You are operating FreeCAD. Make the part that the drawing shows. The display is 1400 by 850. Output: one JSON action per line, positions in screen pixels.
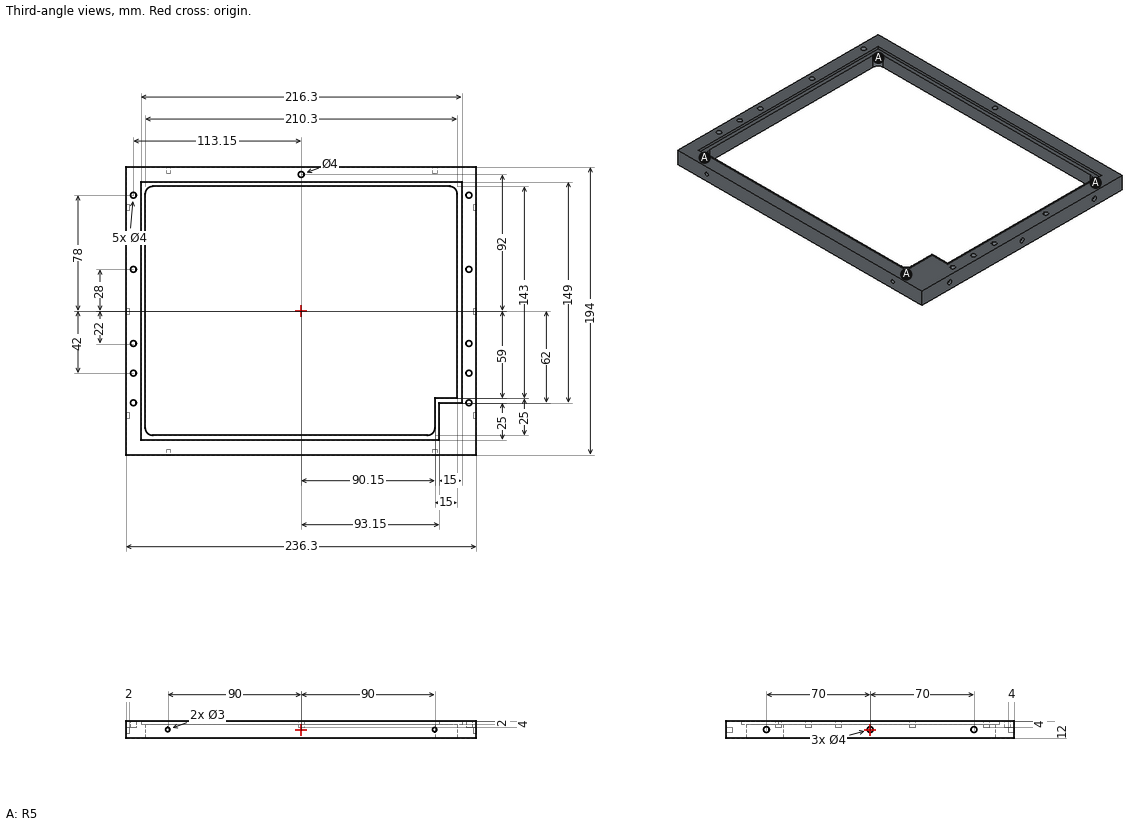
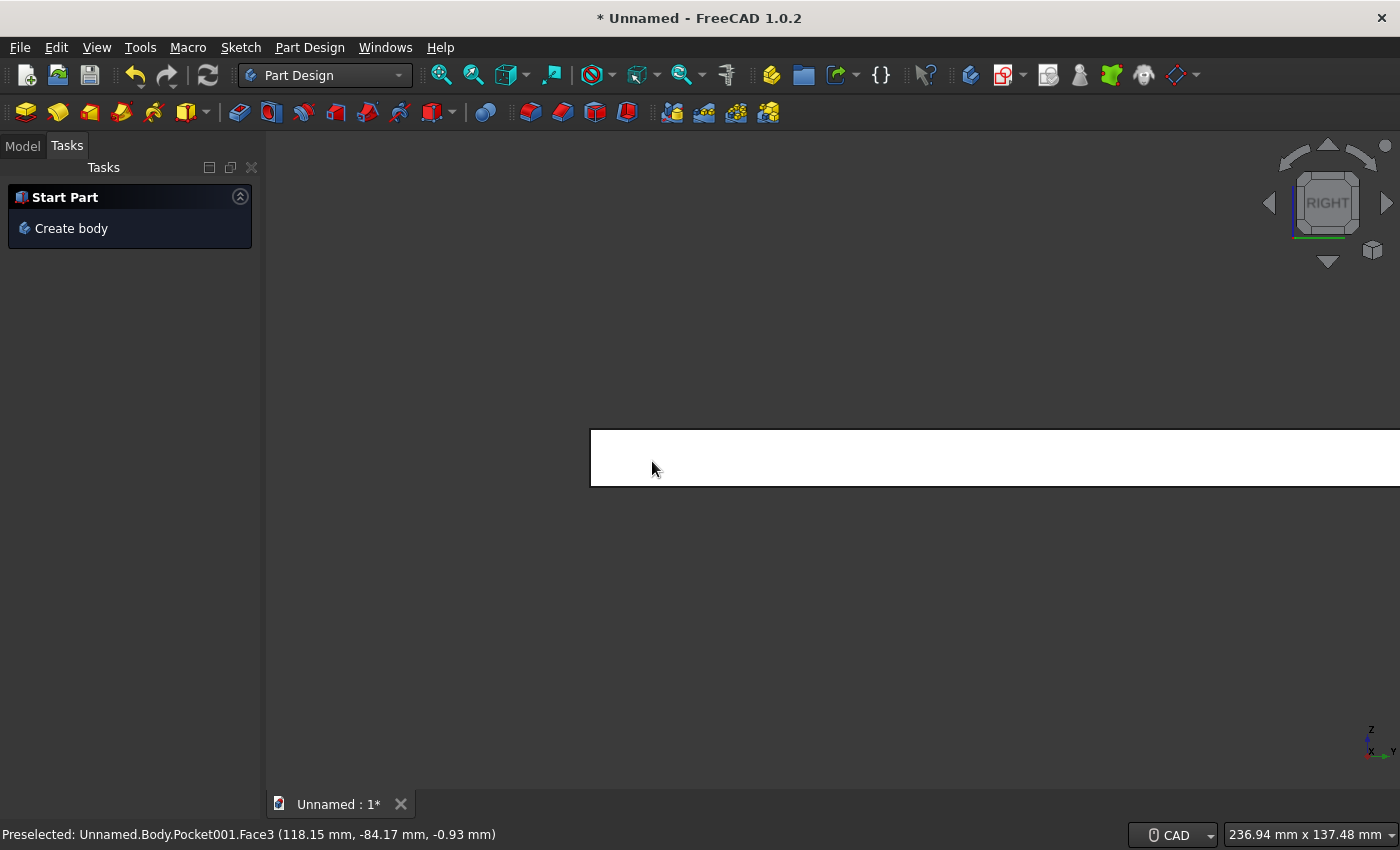
{"action": "left_click", "coordinate": [442, 76]}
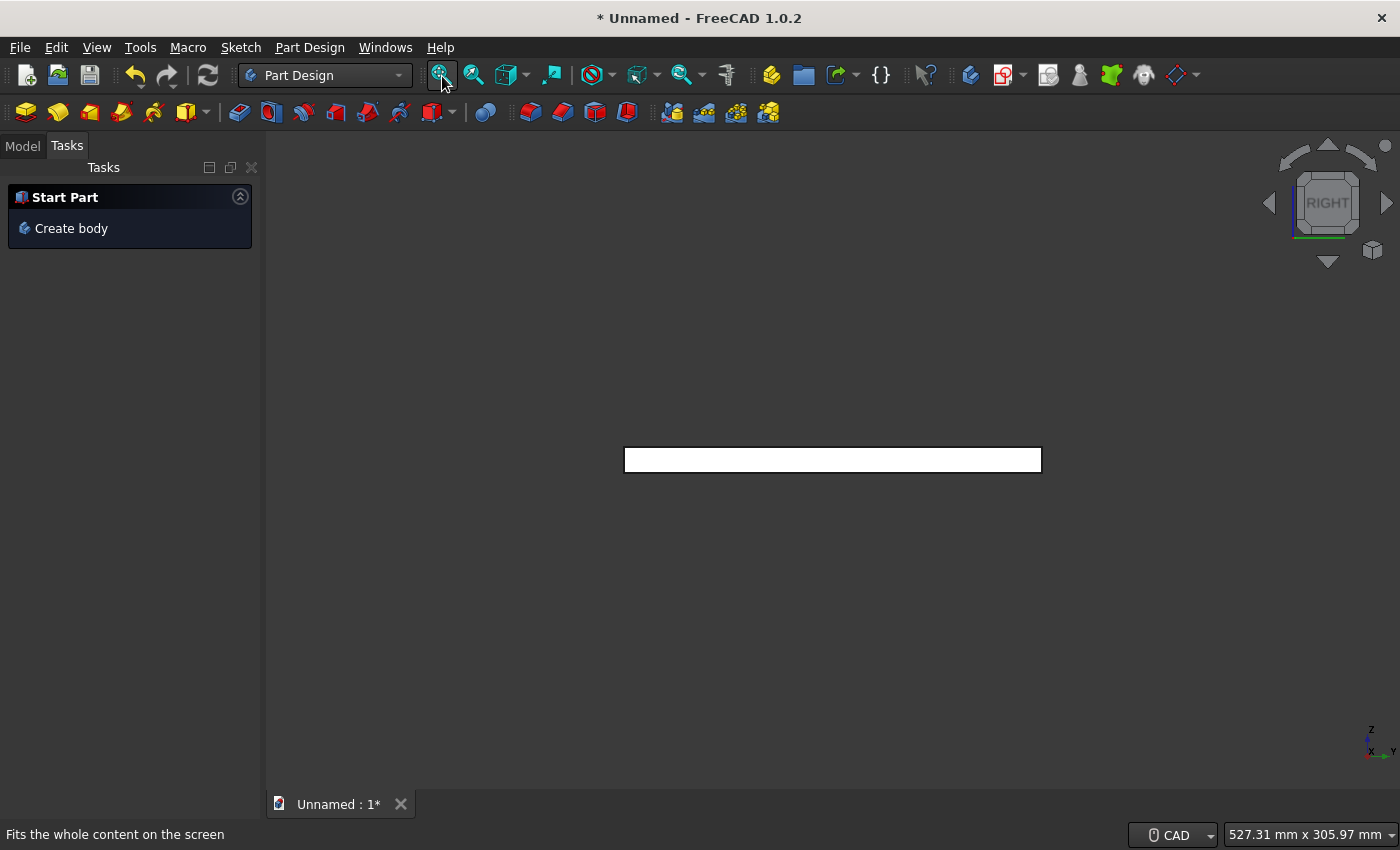
{"action": "key", "text": "5"}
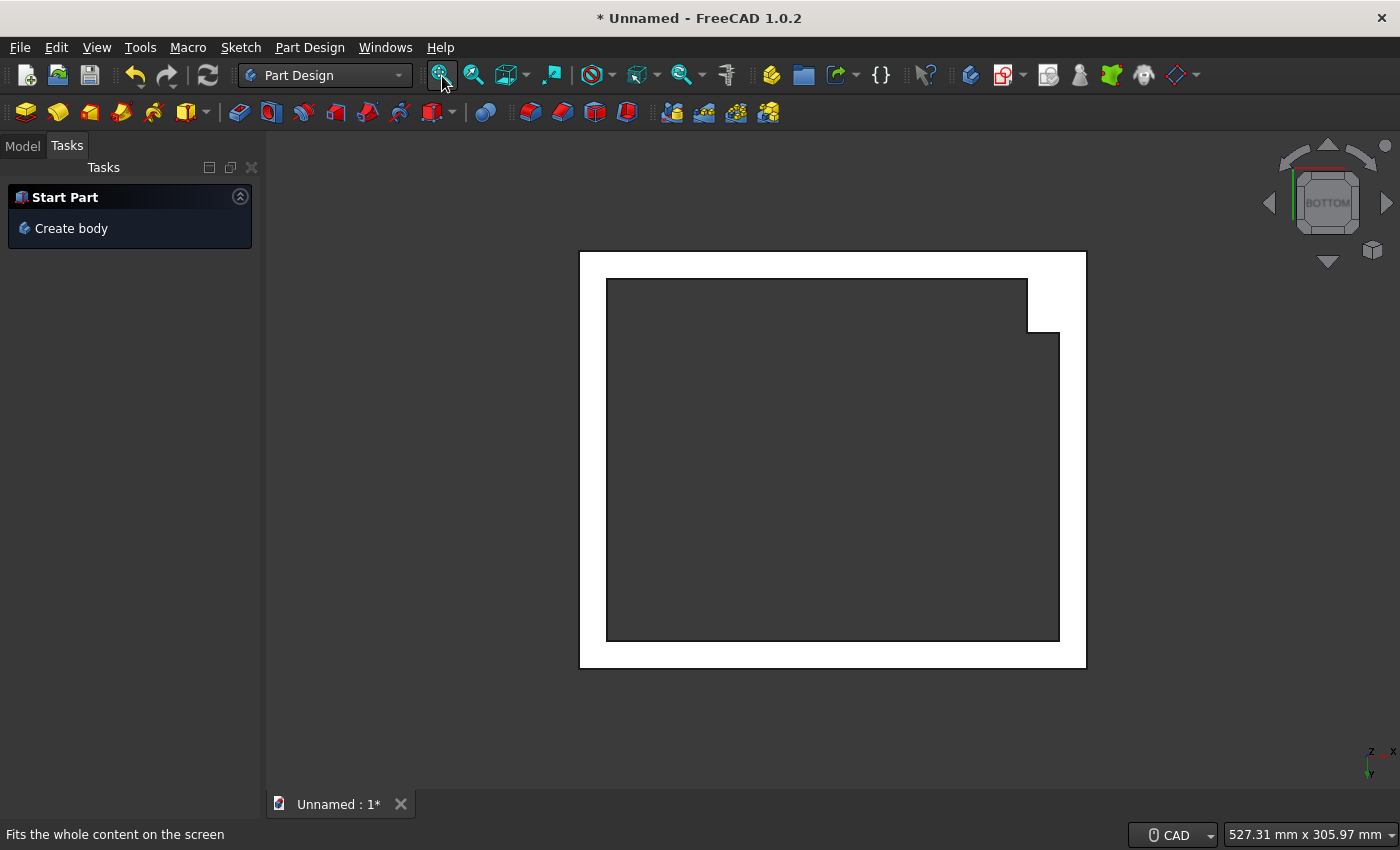
{"action": "scroll", "coordinate": [1027, 278], "scroll_direction": "up", "scroll_amount": 4}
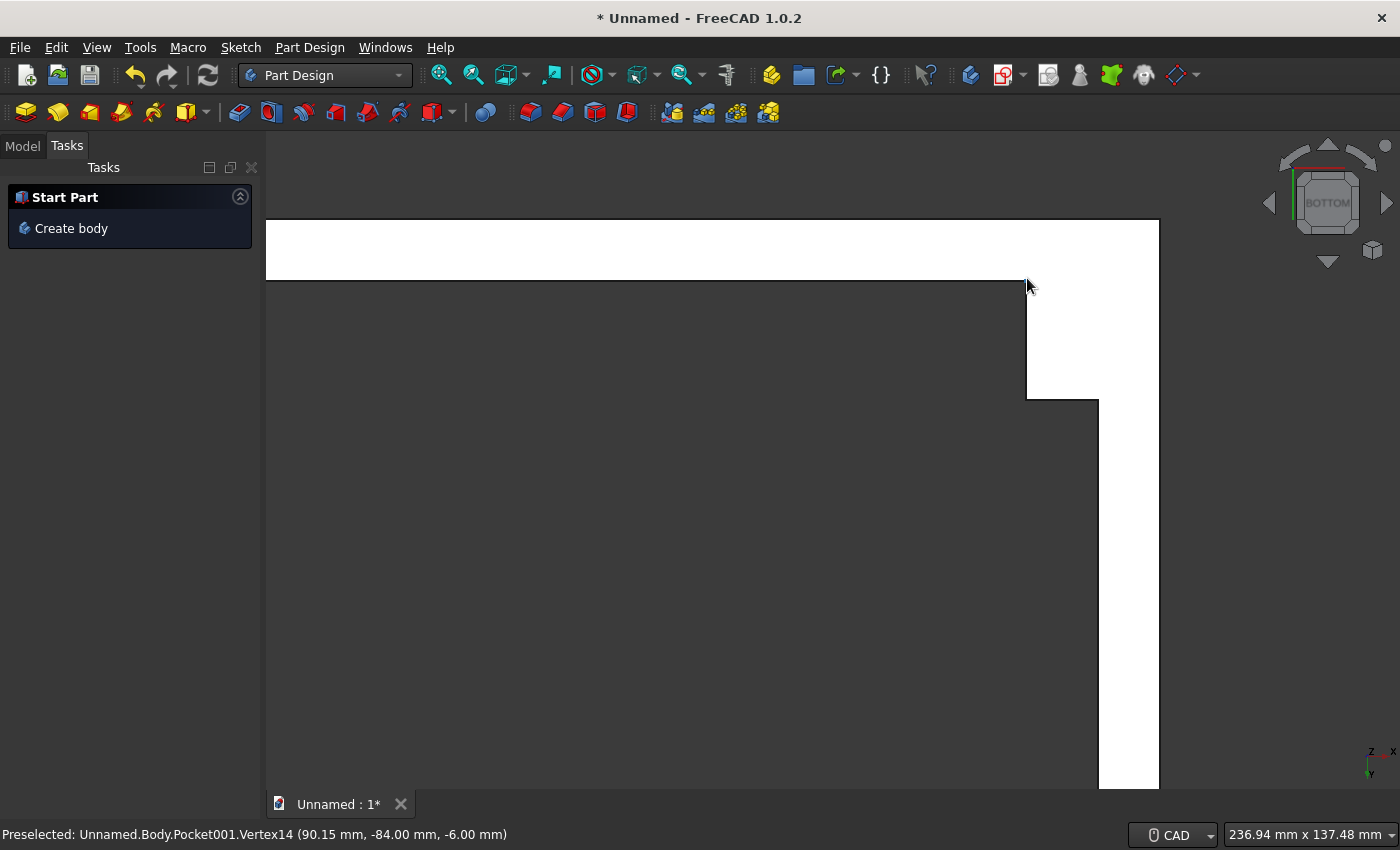
{"action": "left_click", "coordinate": [442, 76]}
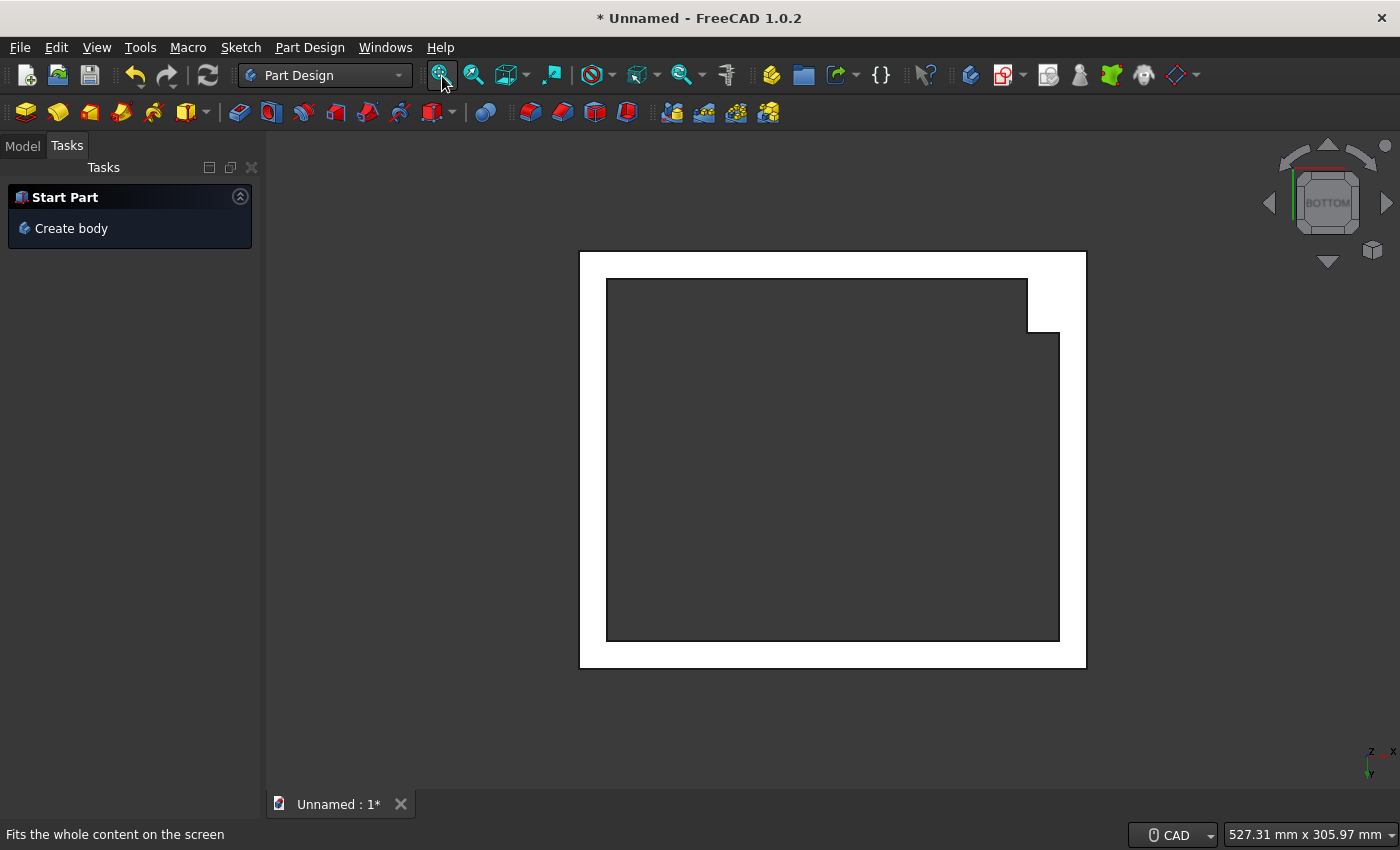
{"action": "key", "text": "4"}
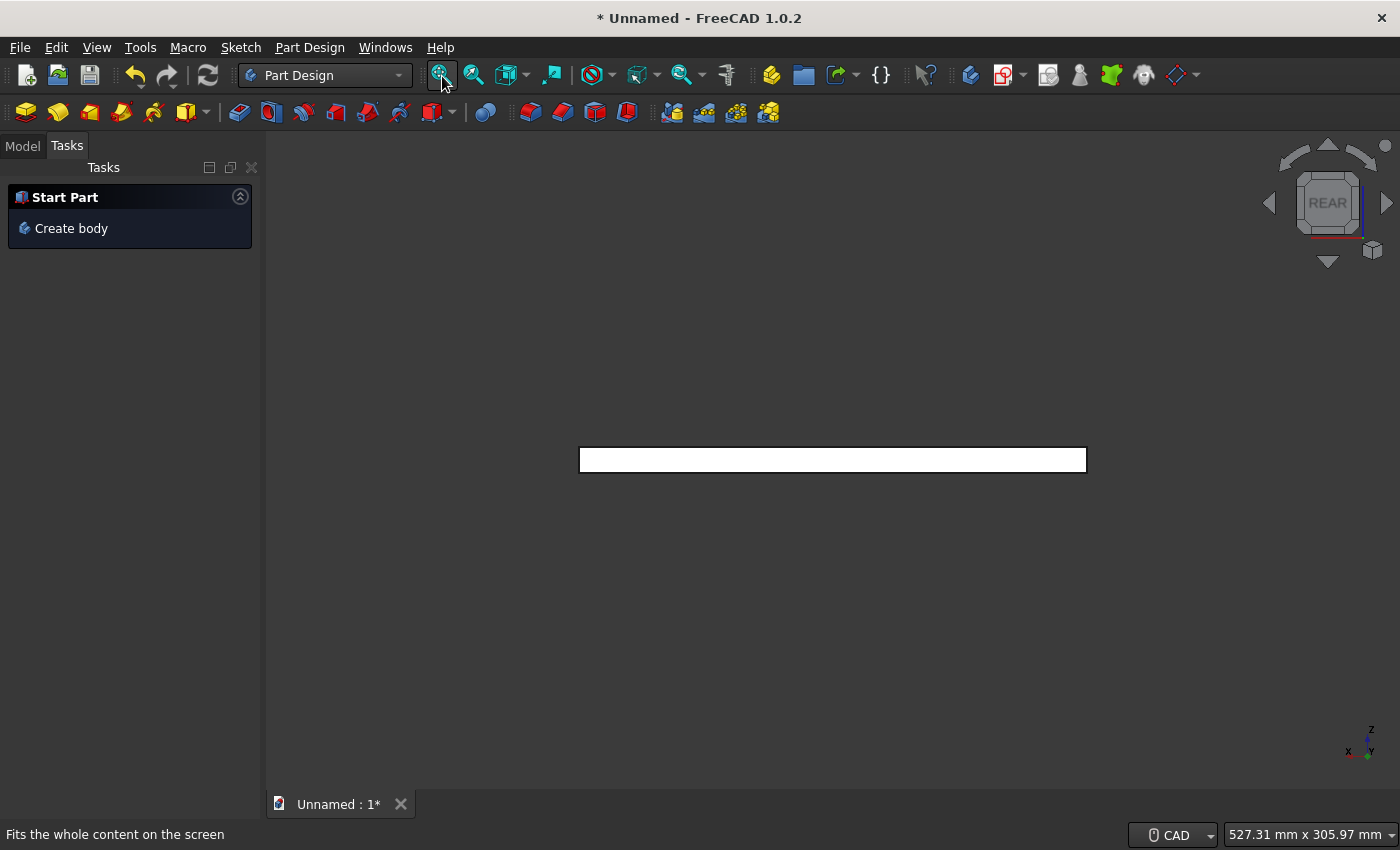
{"action": "left_click", "coordinate": [442, 76]}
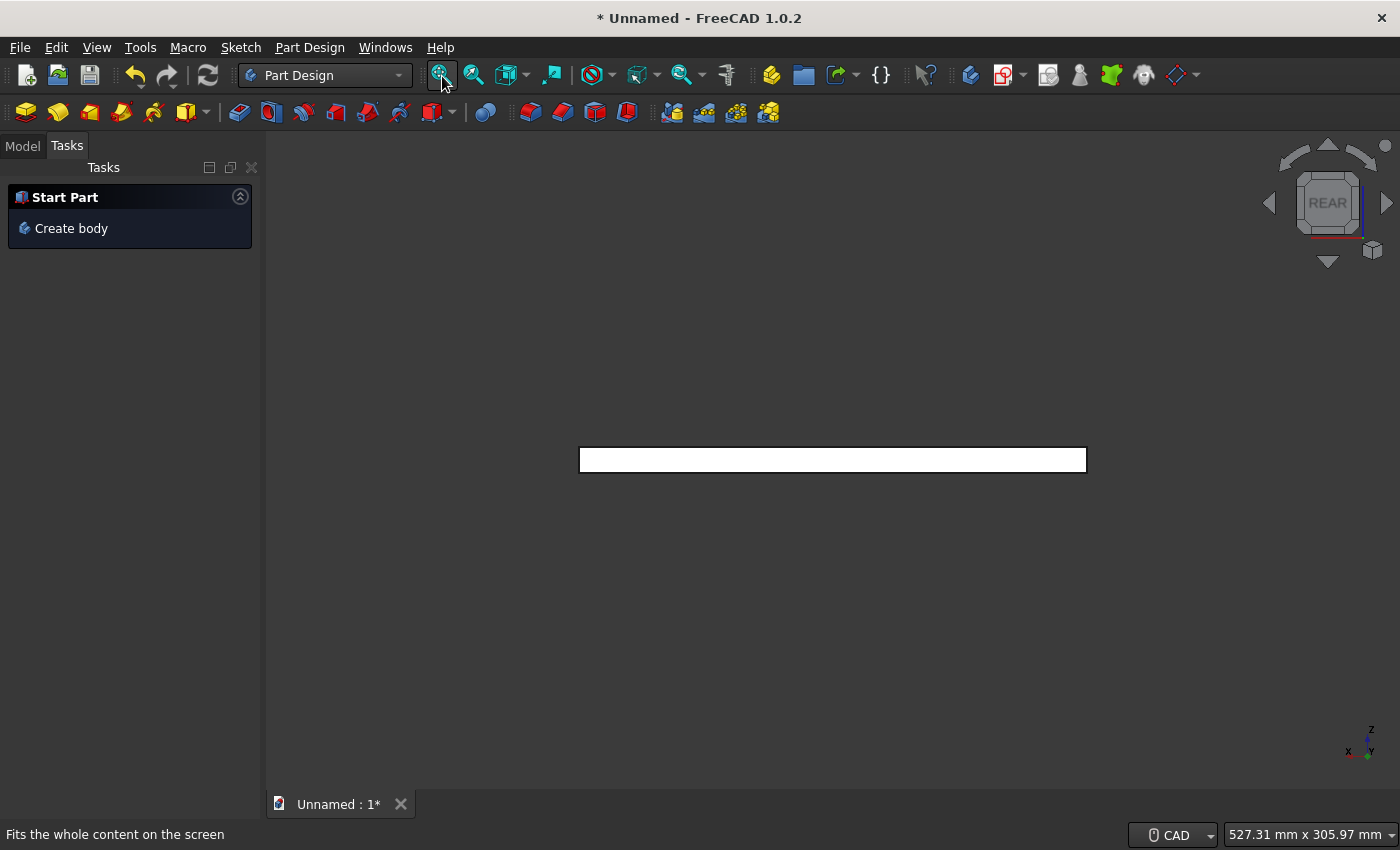
{"action": "scroll", "coordinate": [639, 461], "scroll_direction": "up", "scroll_amount": 4}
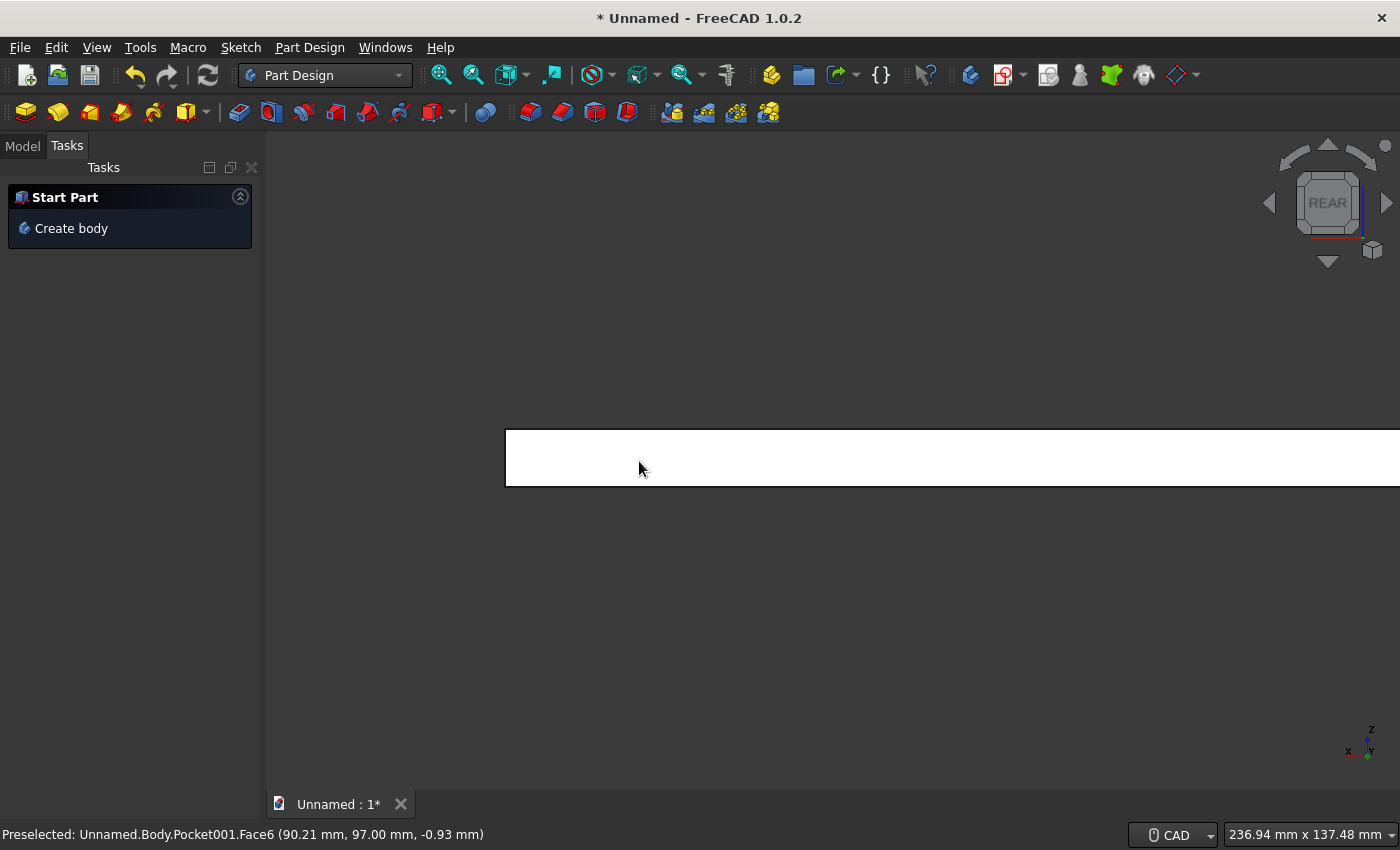
{"action": "left_click", "coordinate": [442, 76]}